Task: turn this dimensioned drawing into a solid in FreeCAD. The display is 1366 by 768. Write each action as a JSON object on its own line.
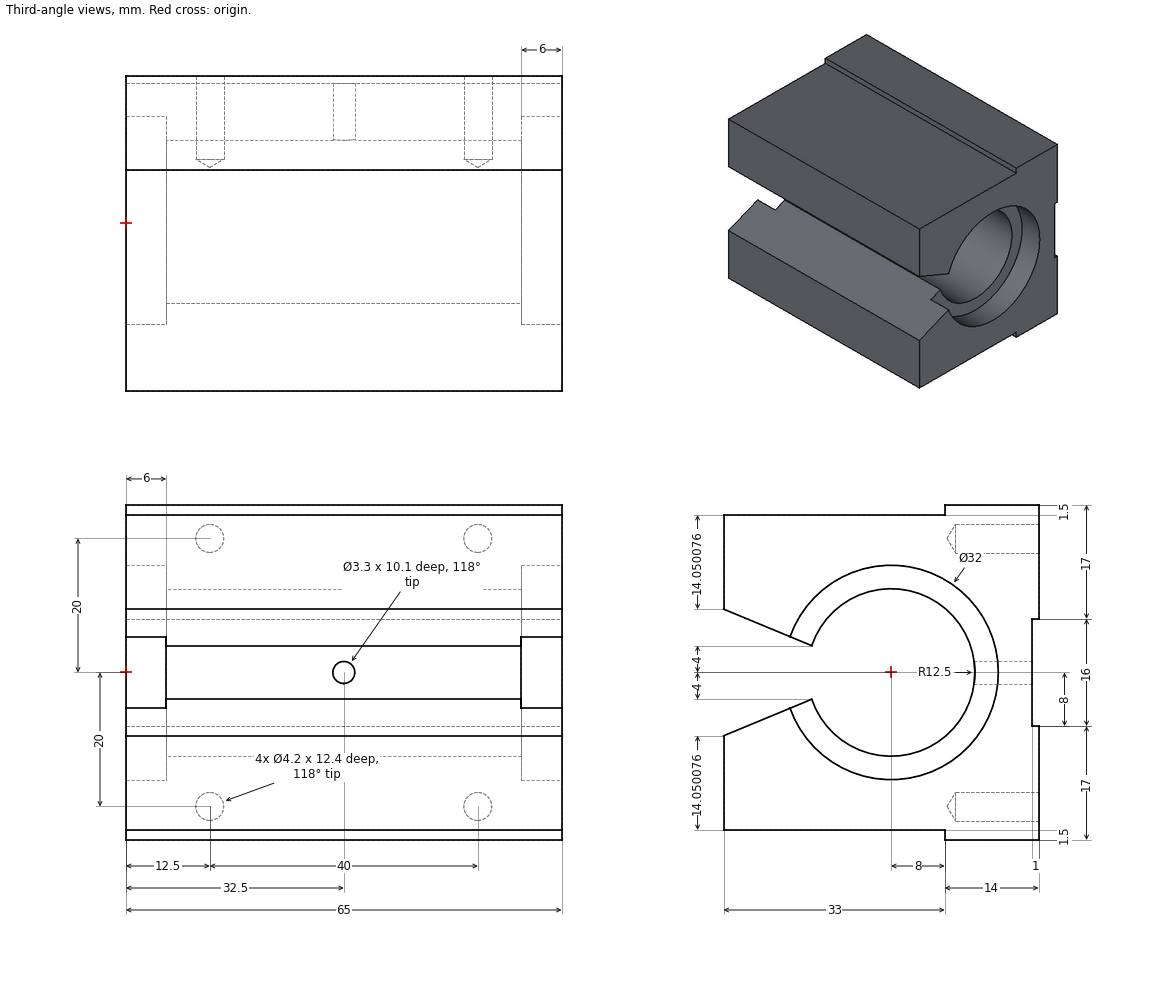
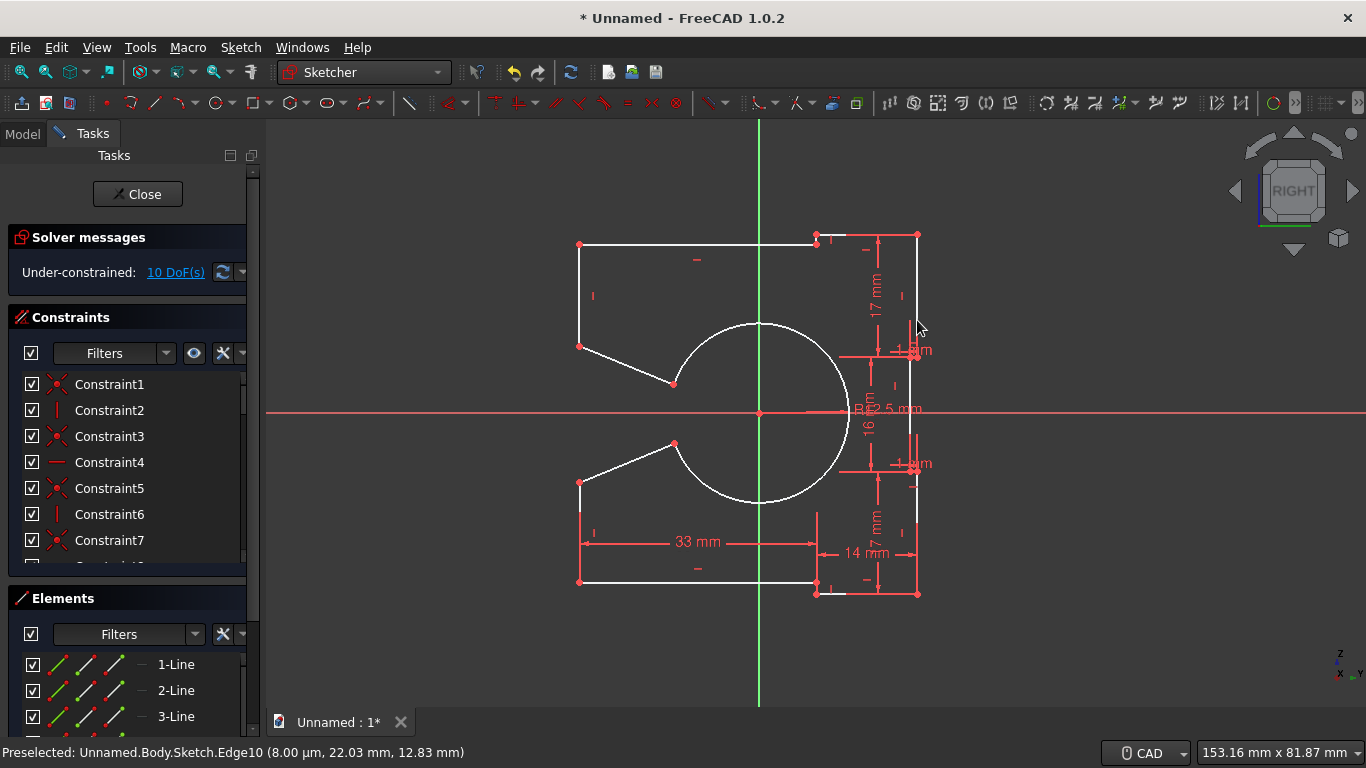
{"action": "left_click", "coordinate": [887, 235]}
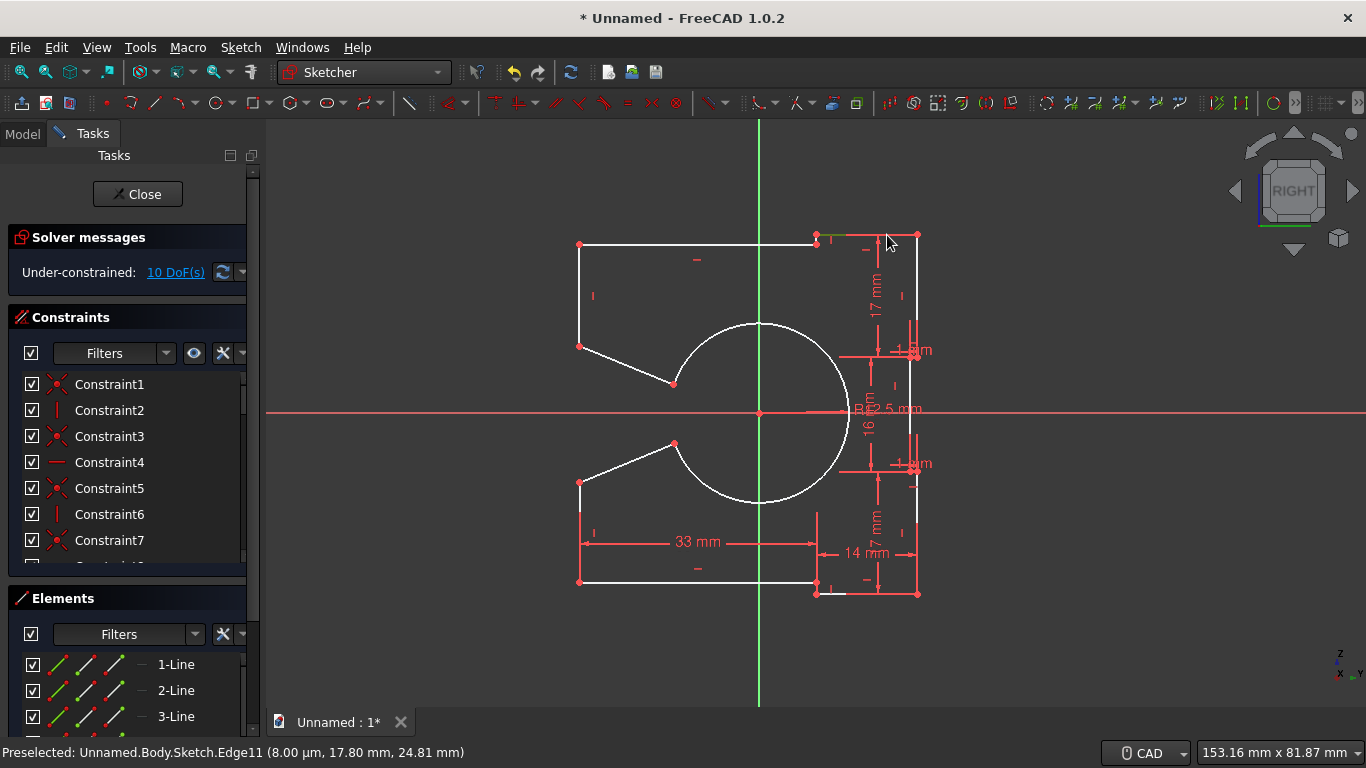
{"action": "key", "text": "l"}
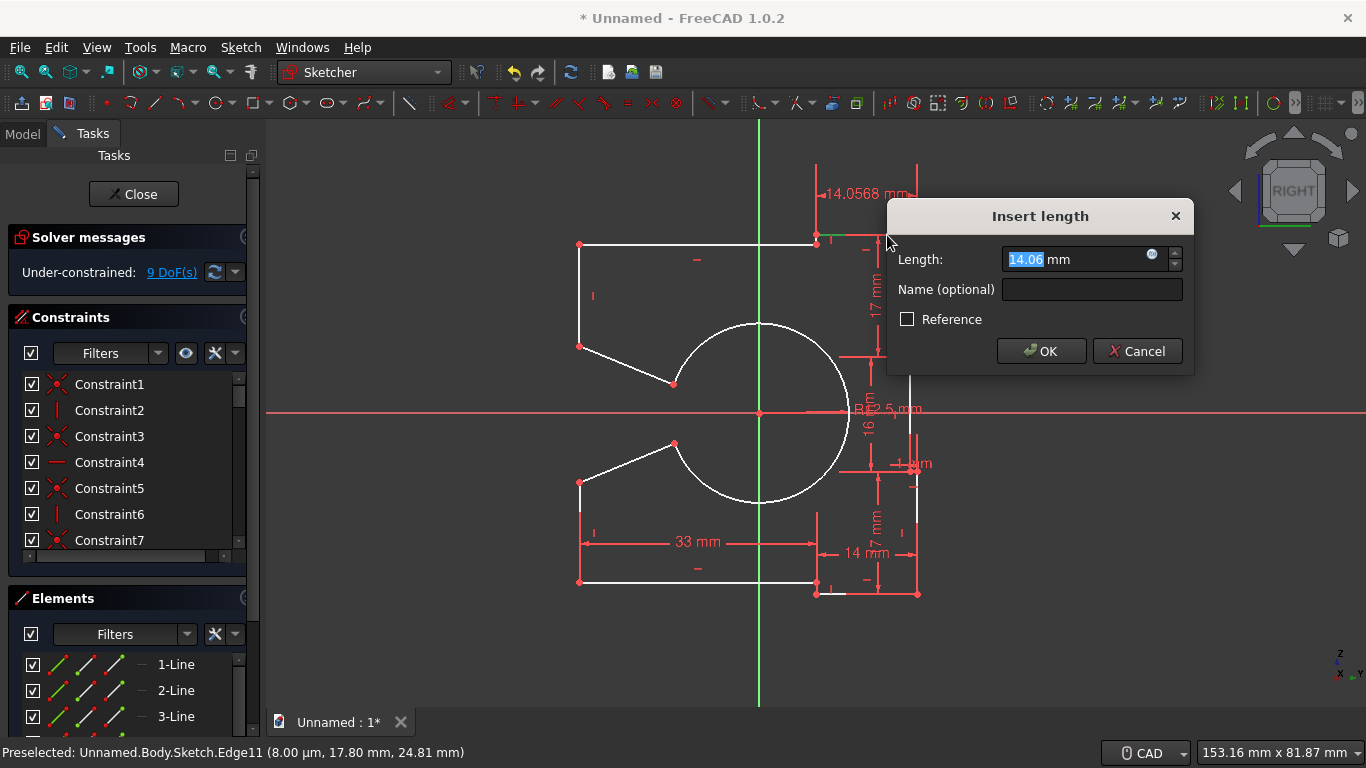
{"action": "type", "text": "14"}
{"action": "key", "text": "Return"}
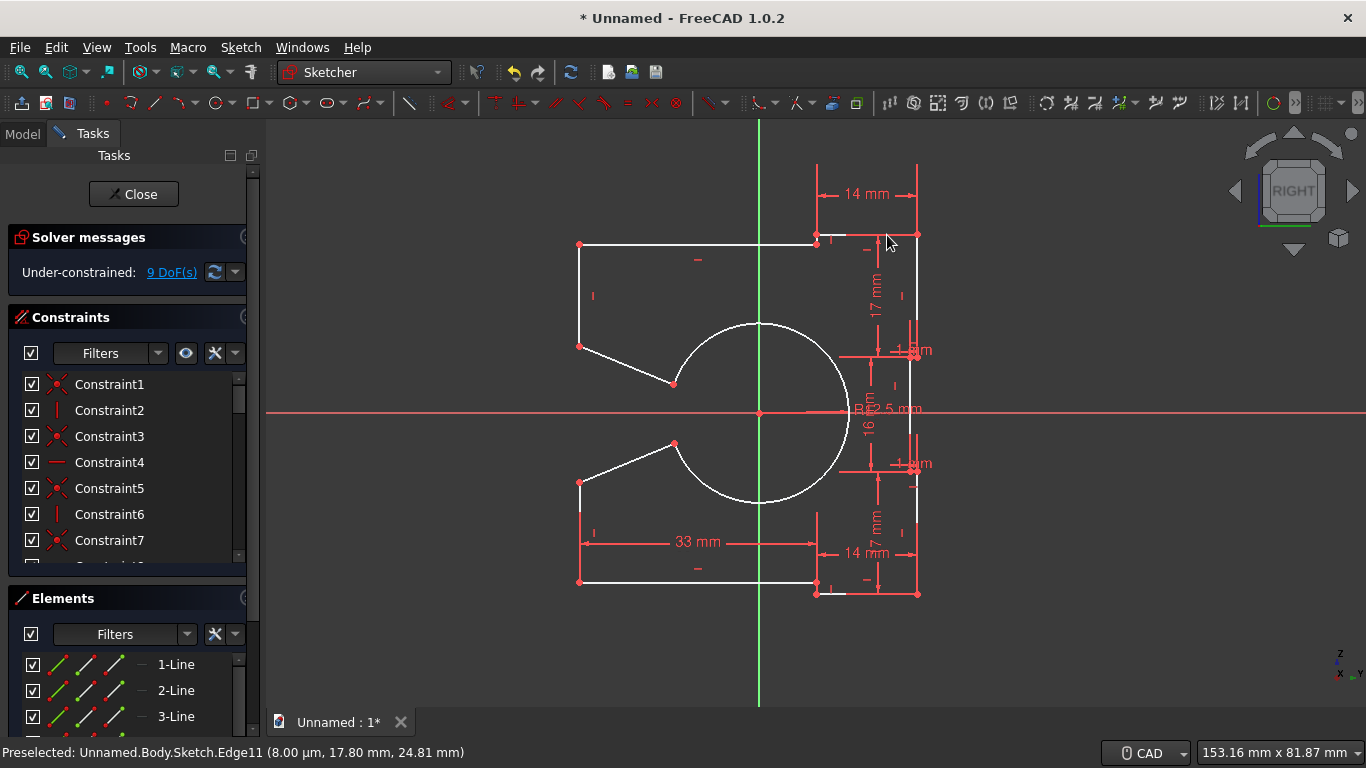
{"action": "left_click", "coordinate": [746, 245]}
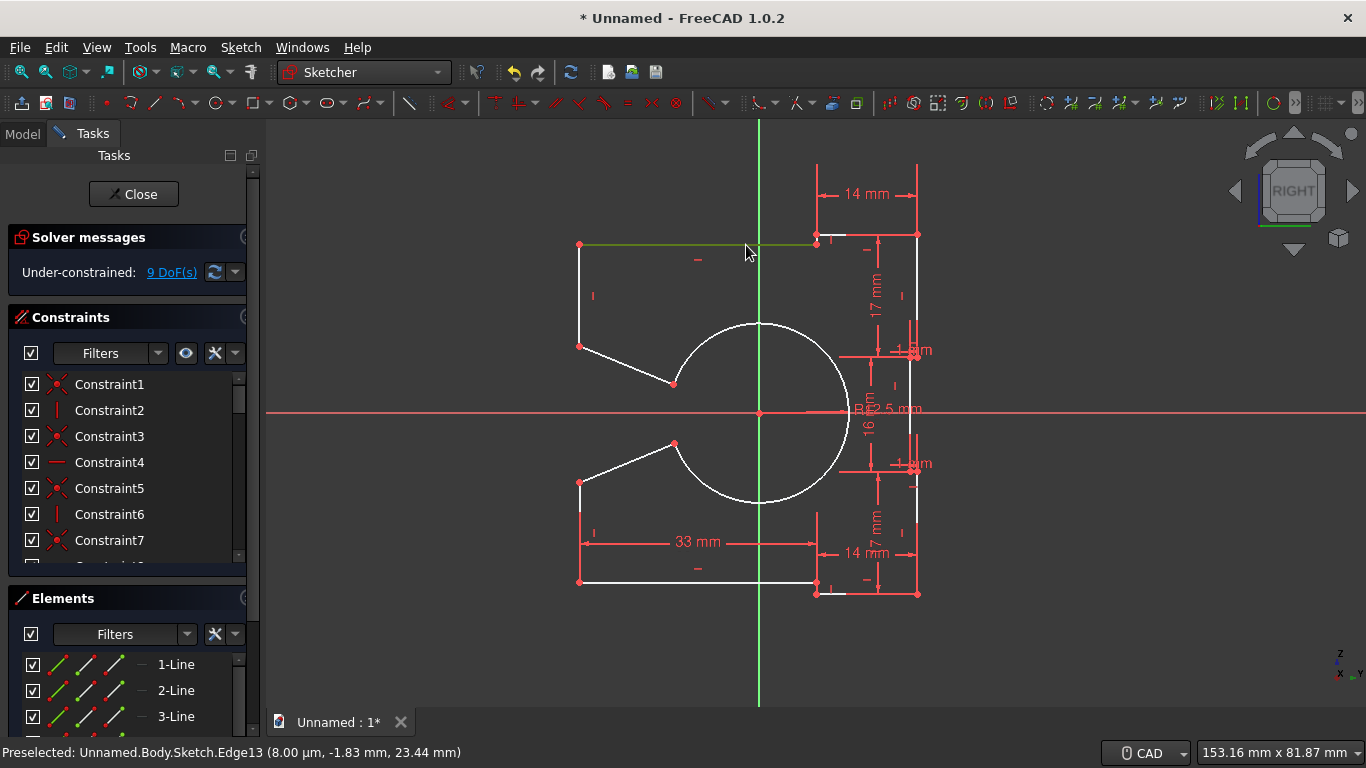
{"action": "key", "text": "l"}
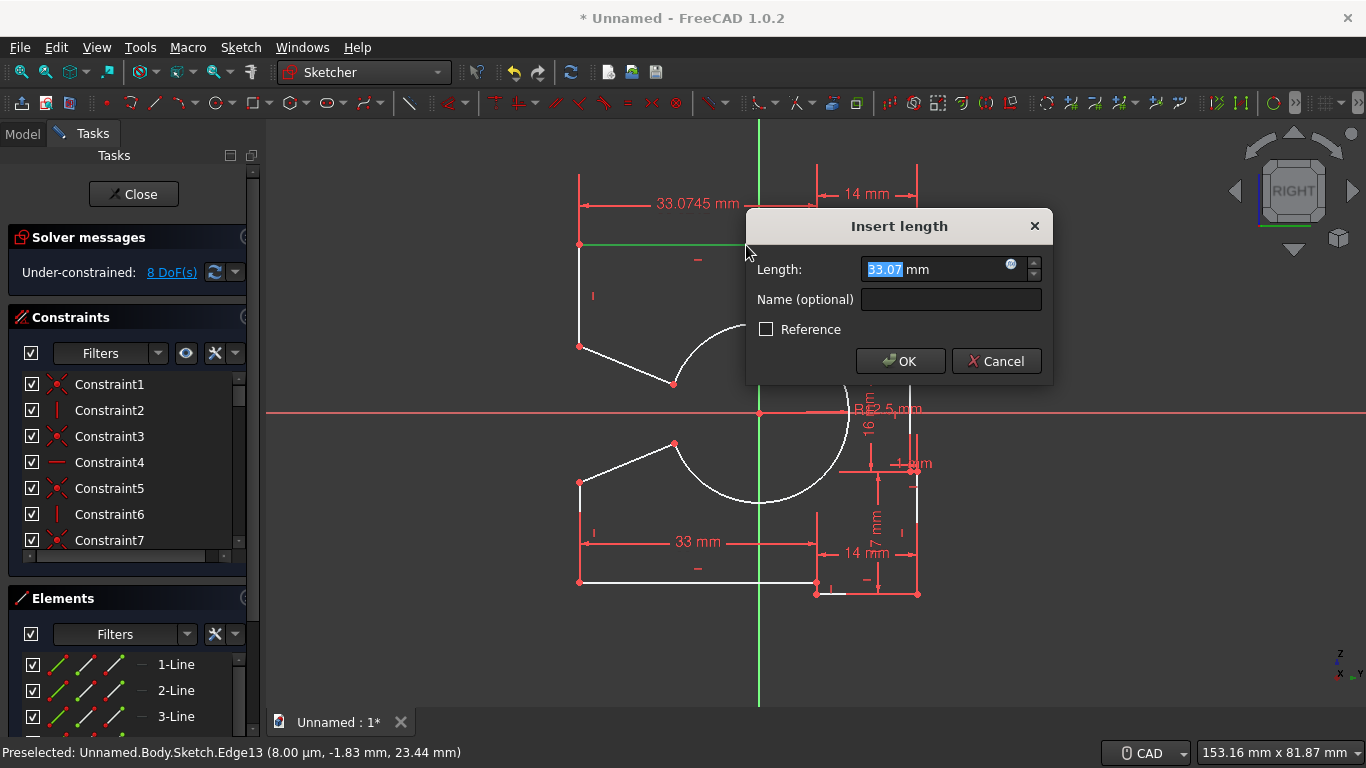
{"action": "type", "text": "33"}
{"action": "key", "text": "Return"}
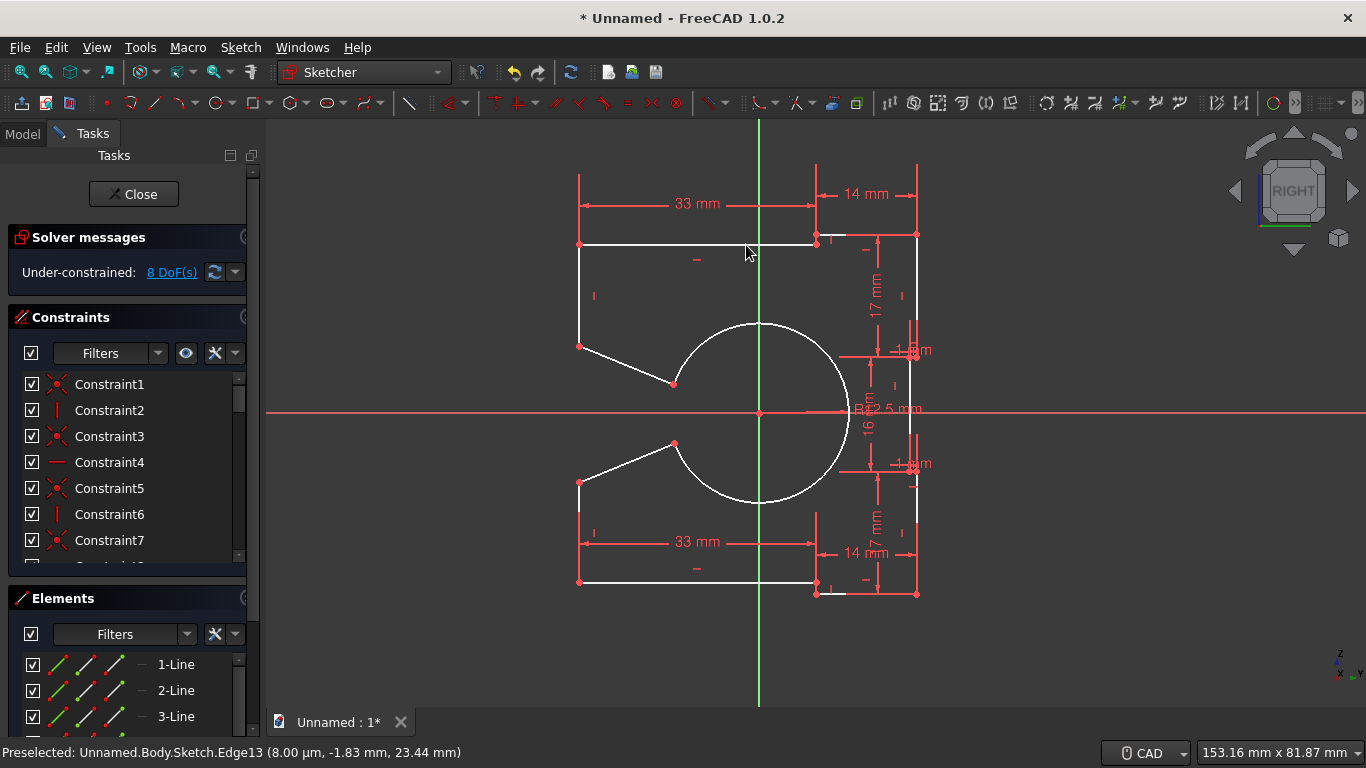
{"action": "scroll", "coordinate": [675, 444], "scroll_direction": "up", "scroll_amount": 2}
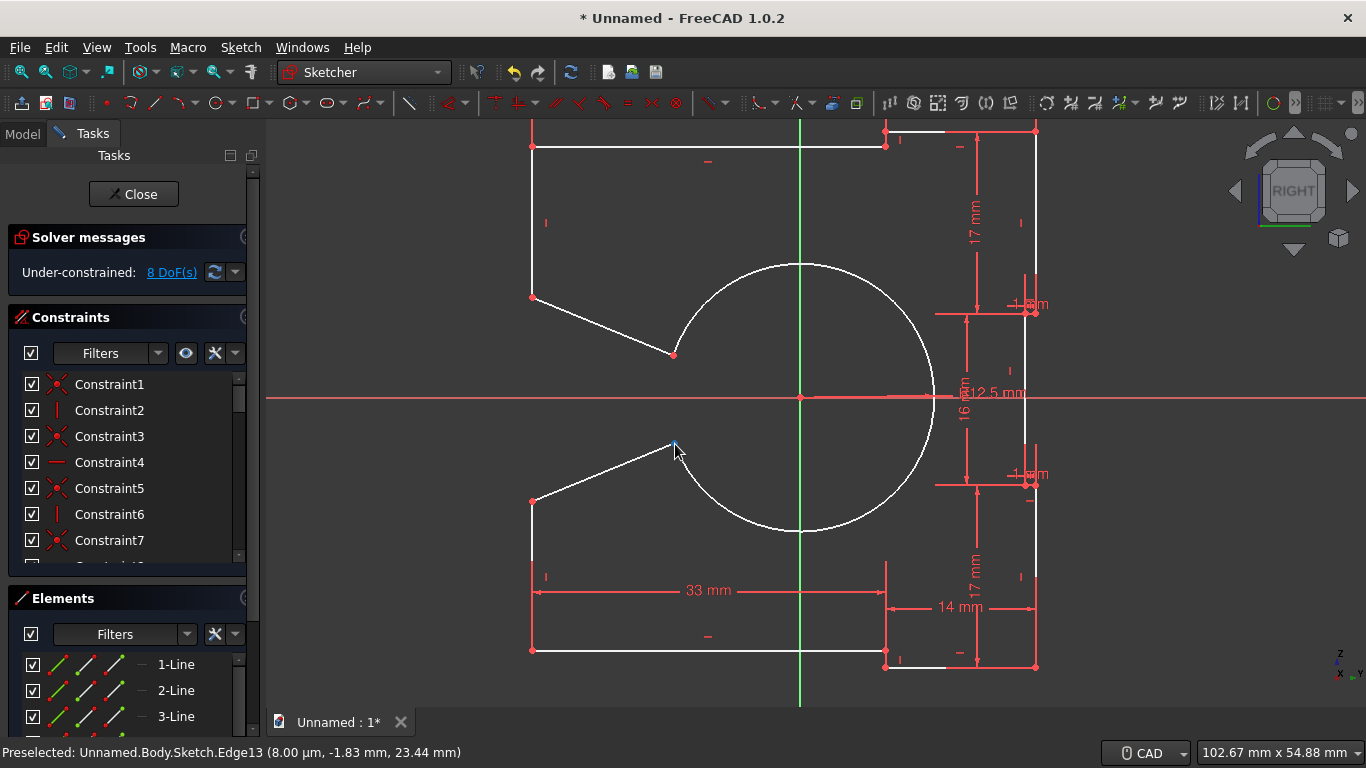
{"action": "left_click", "coordinate": [674, 443]}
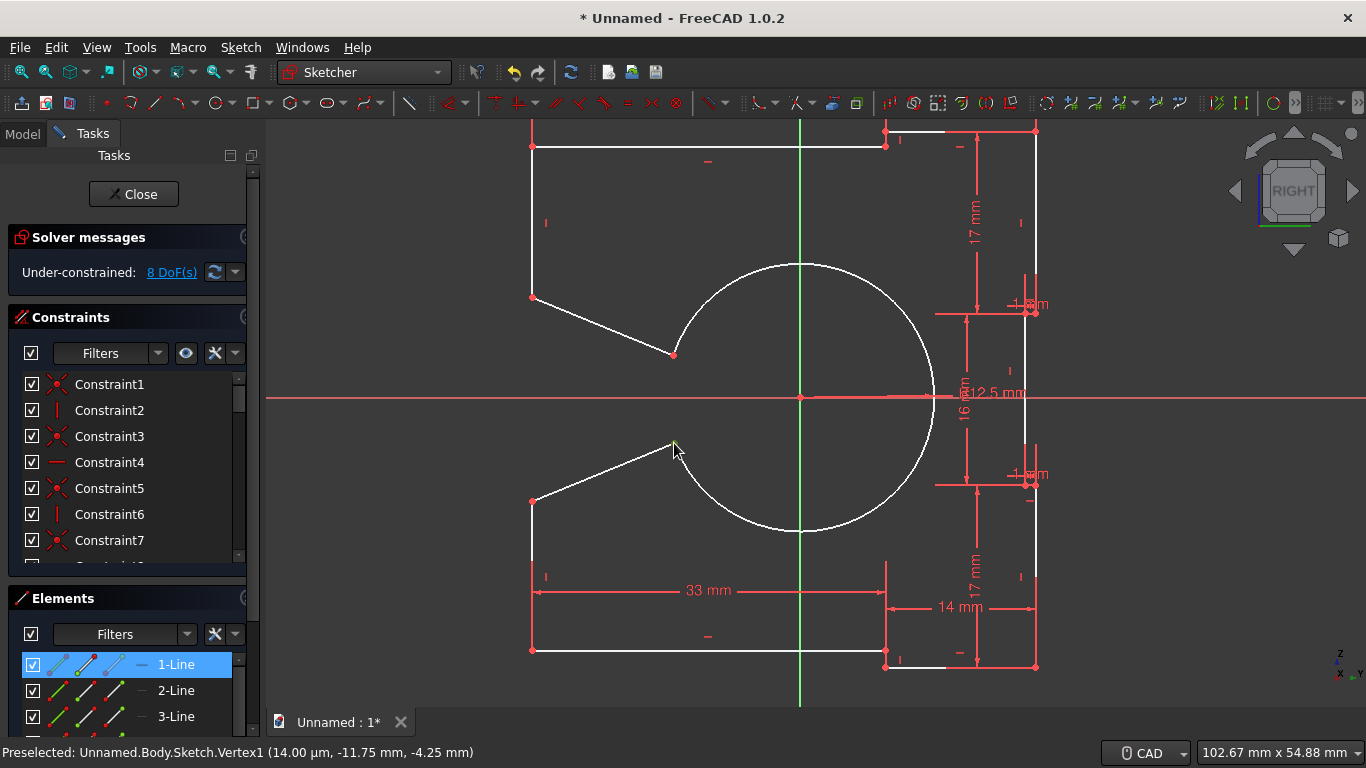
{"action": "key", "text": "i"}